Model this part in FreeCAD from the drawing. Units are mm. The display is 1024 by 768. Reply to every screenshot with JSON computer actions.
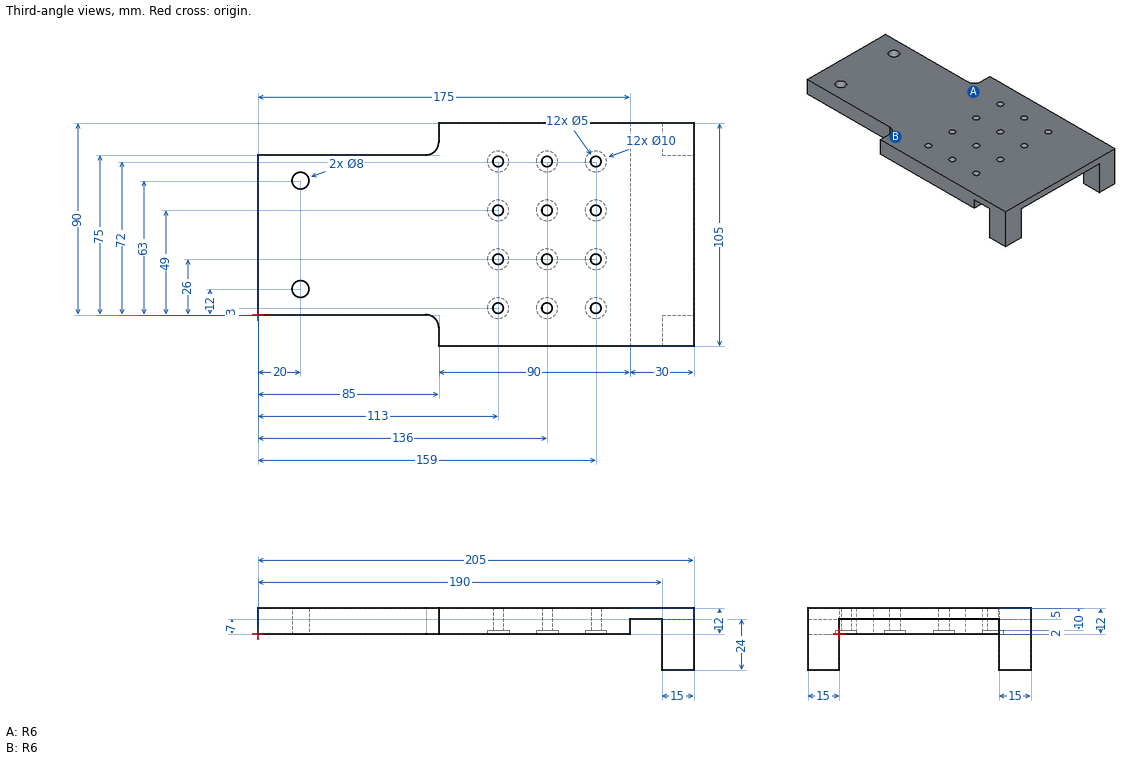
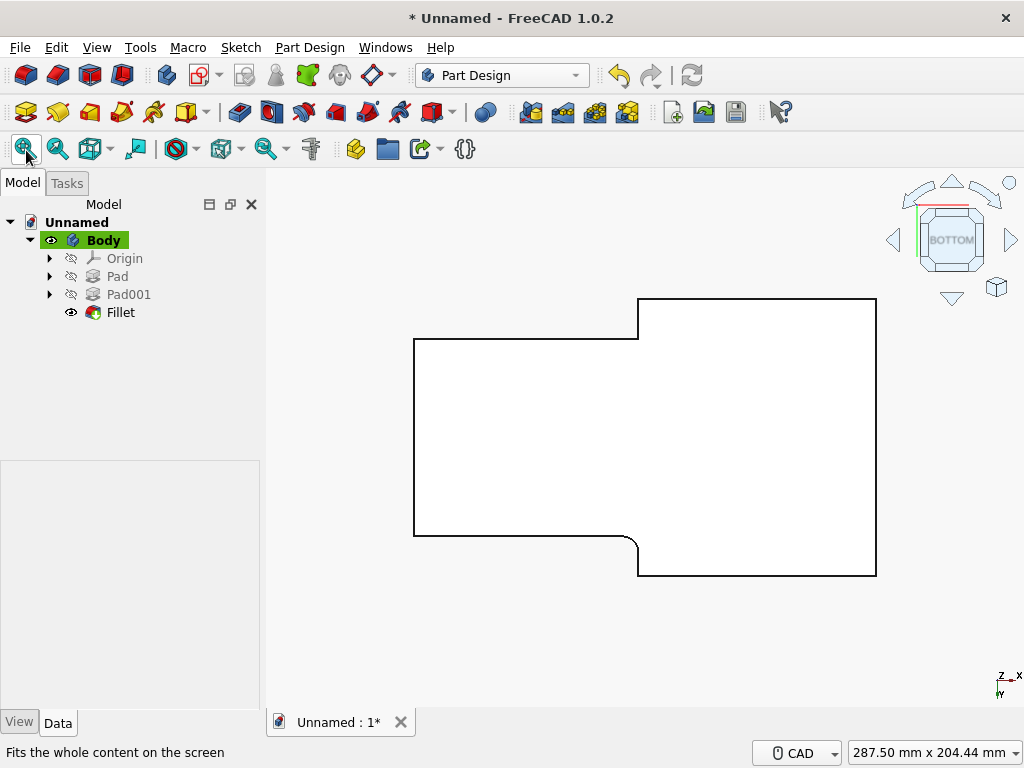
{"action": "key", "text": "4"}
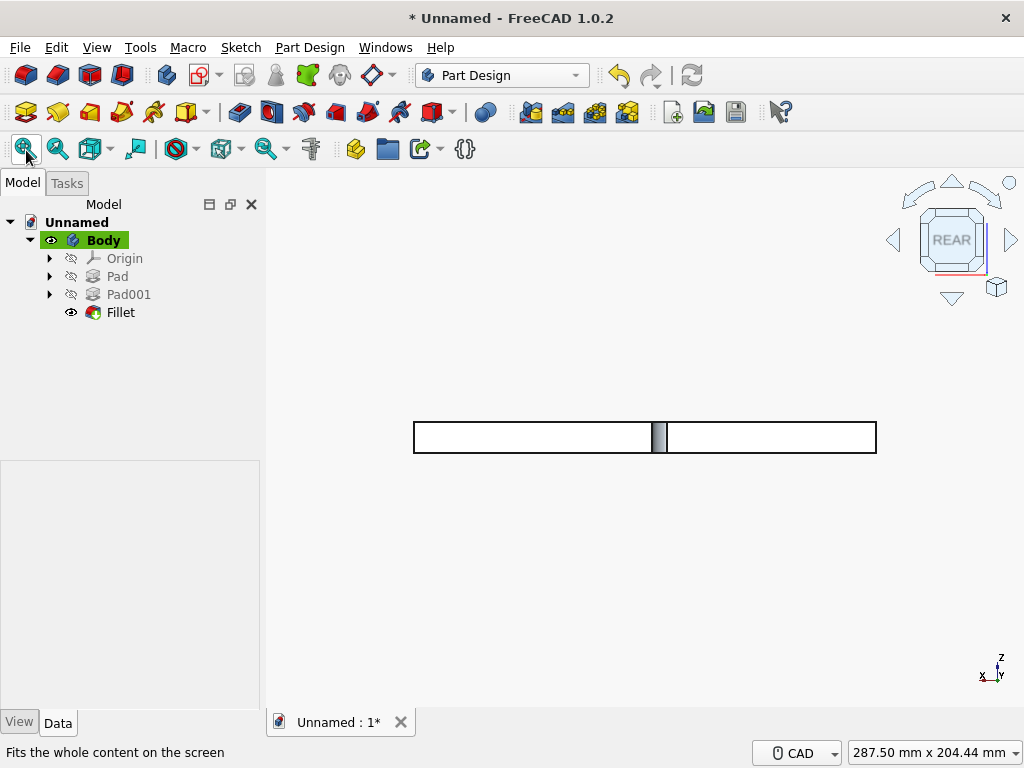
{"action": "key", "text": "6"}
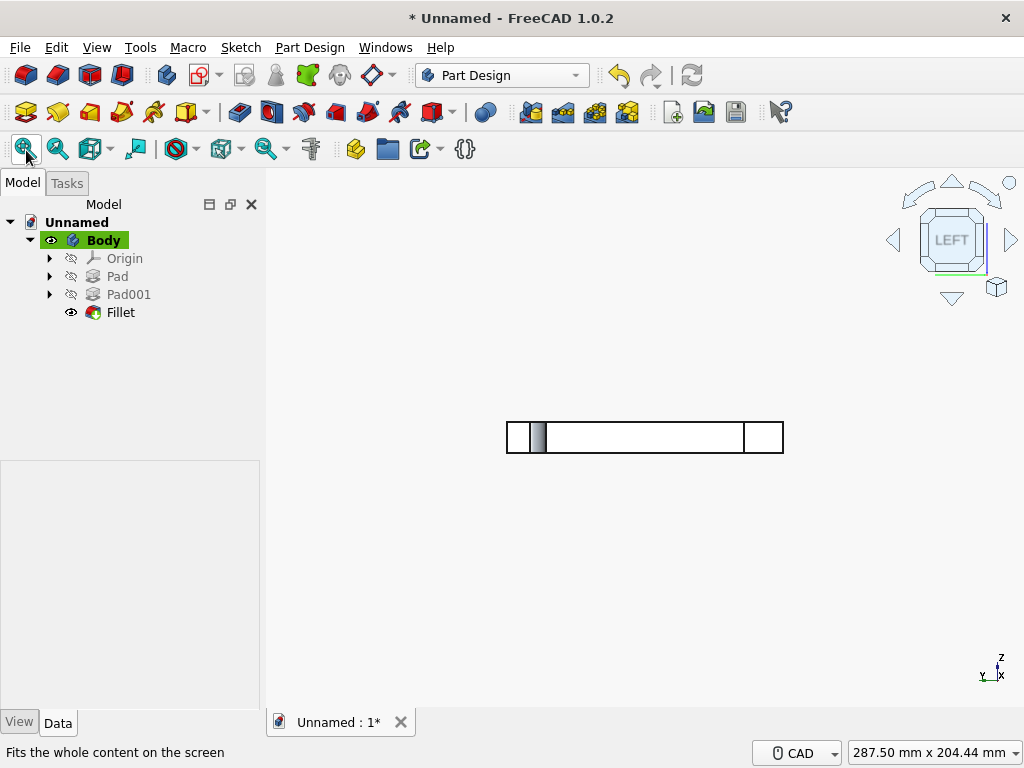
{"action": "left_click", "coordinate": [26, 150]}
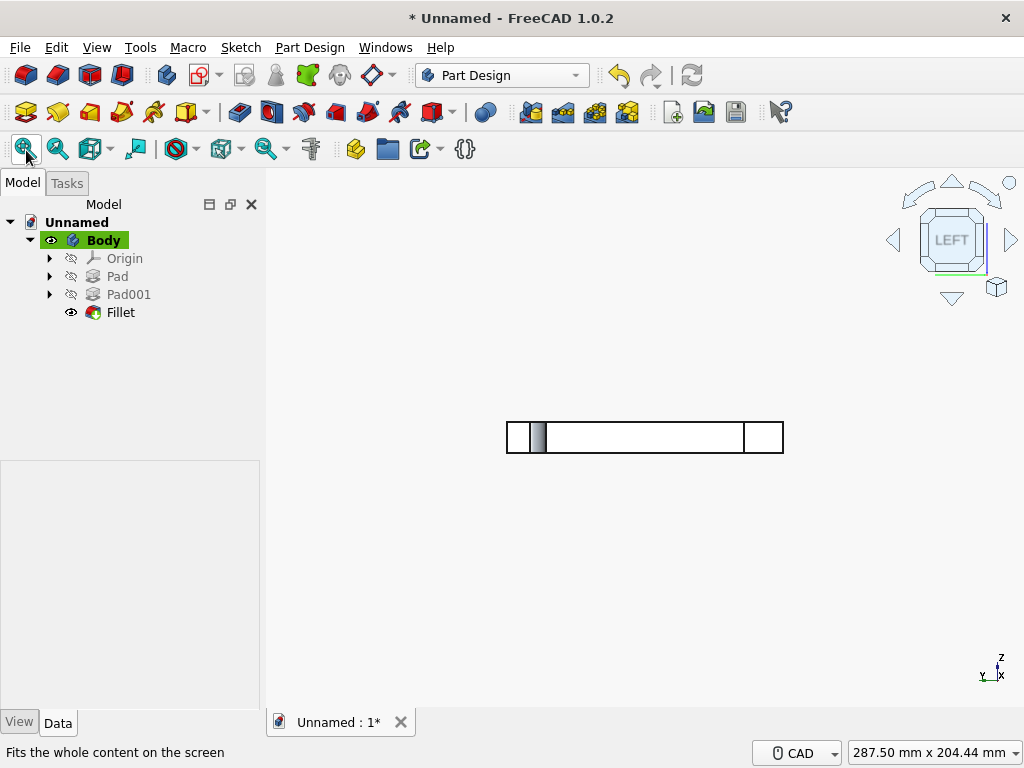
{"action": "key", "text": "v 3"}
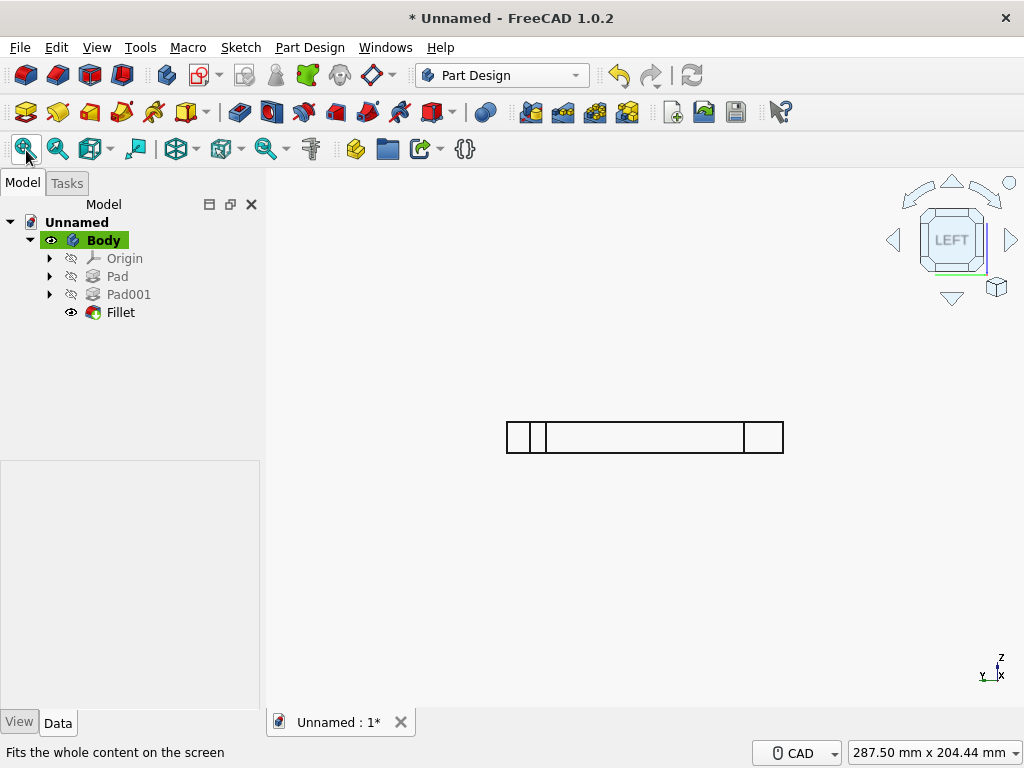
{"action": "key", "text": "0"}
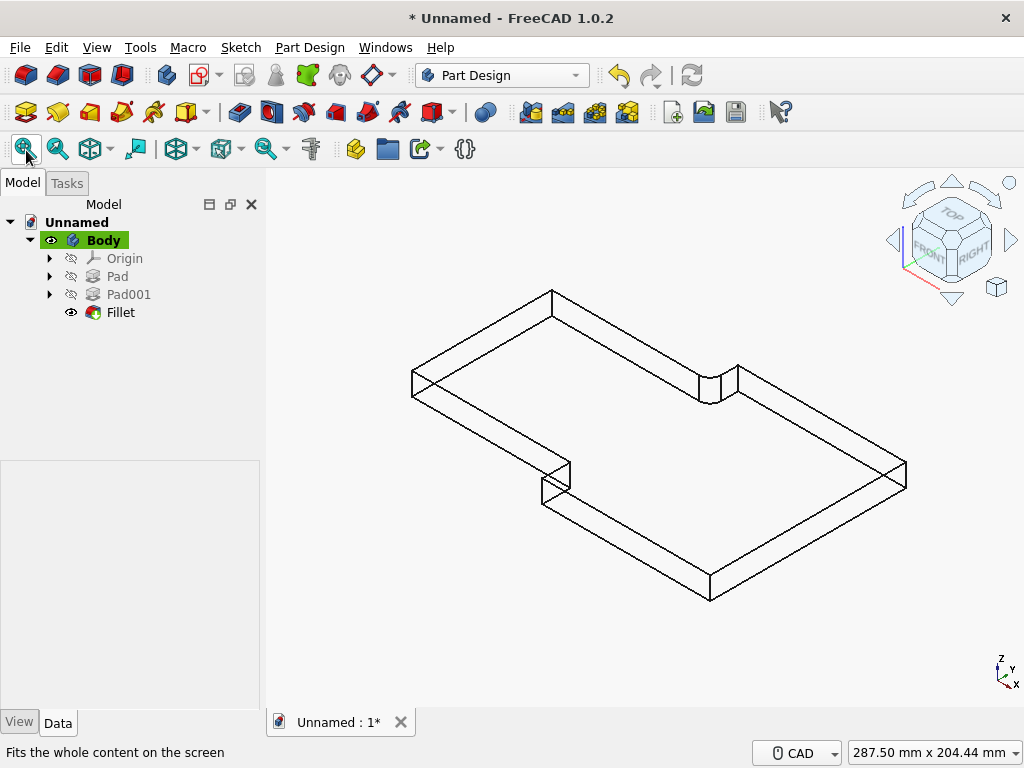
{"action": "left_click", "coordinate": [570, 474]}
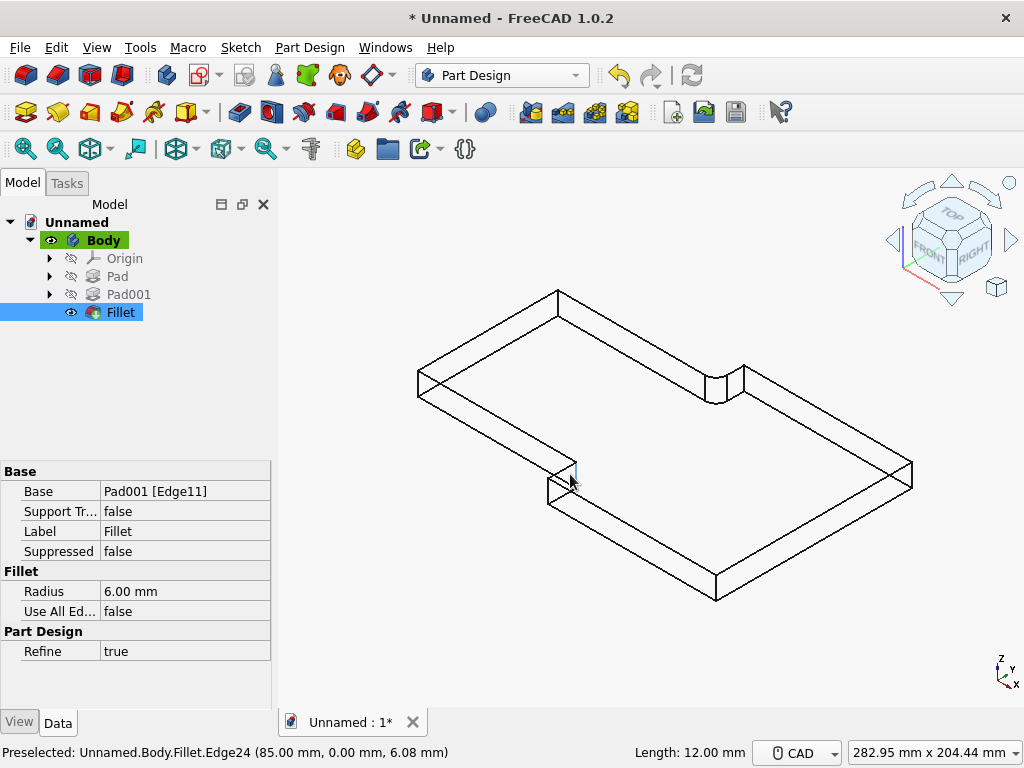
{"action": "key", "text": "v 1"}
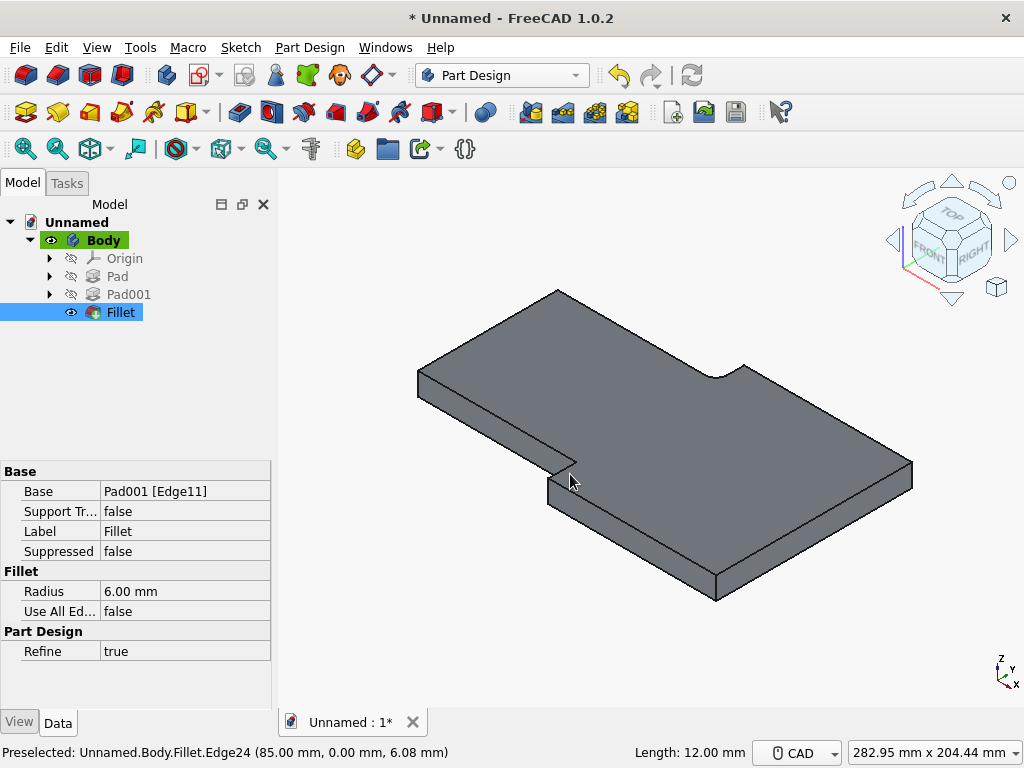
{"action": "left_click", "coordinate": [26, 76]}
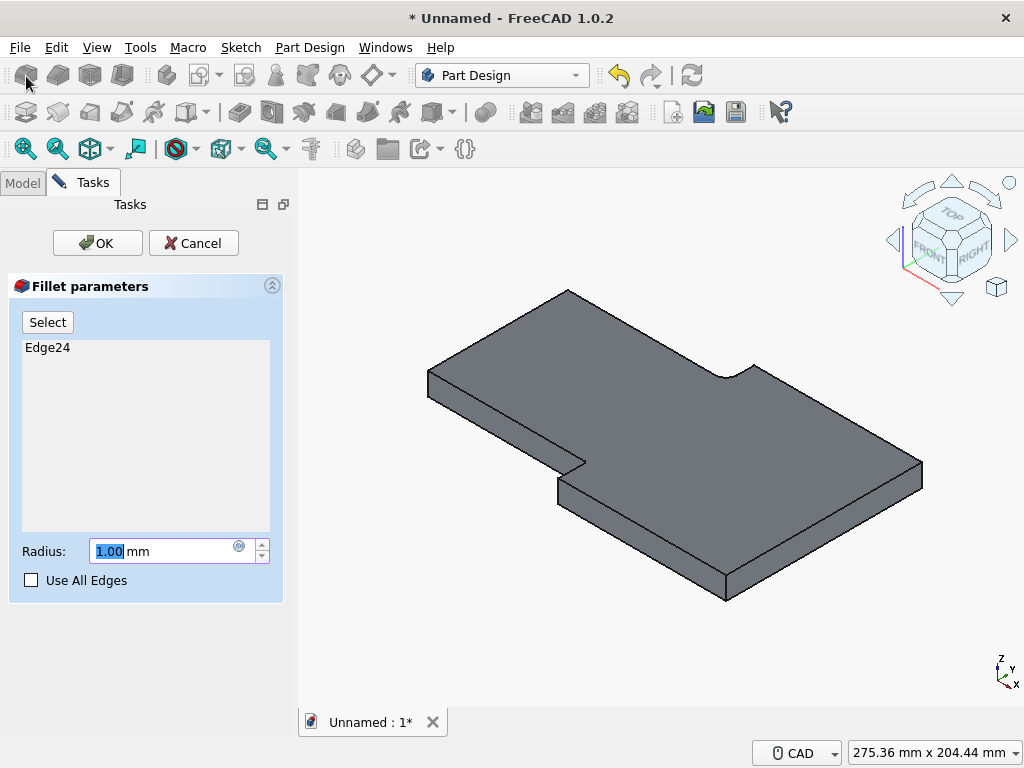
{"action": "type", "text": "6"}
{"action": "key", "text": "Tab"}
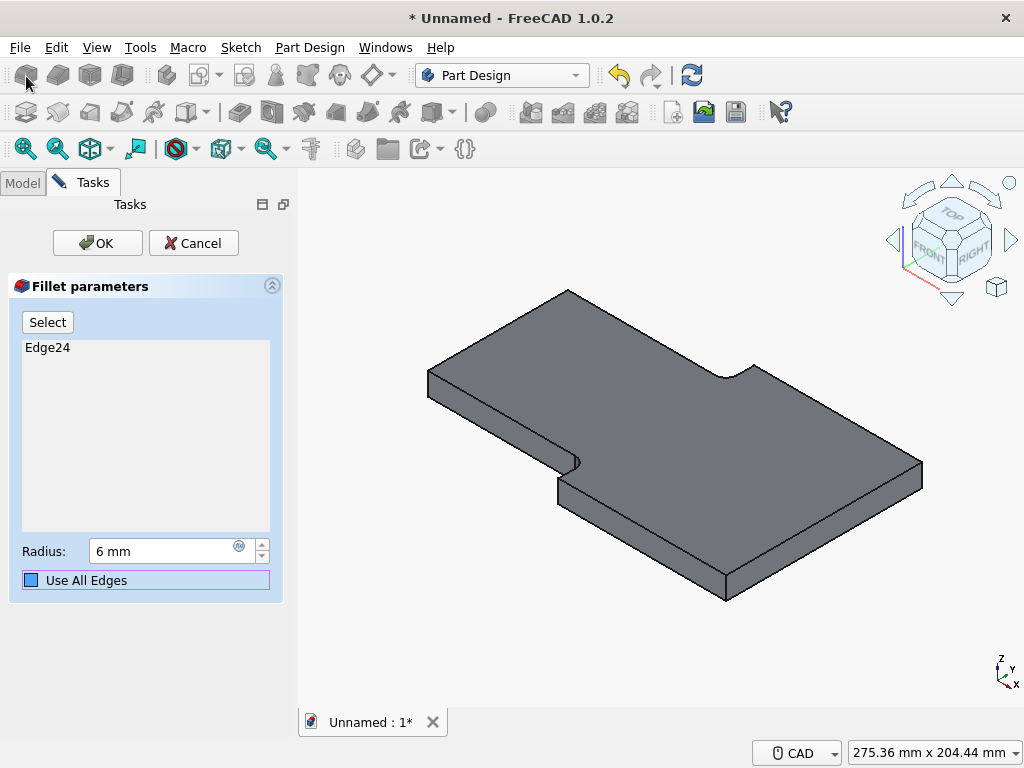
{"action": "left_click", "coordinate": [98, 243]}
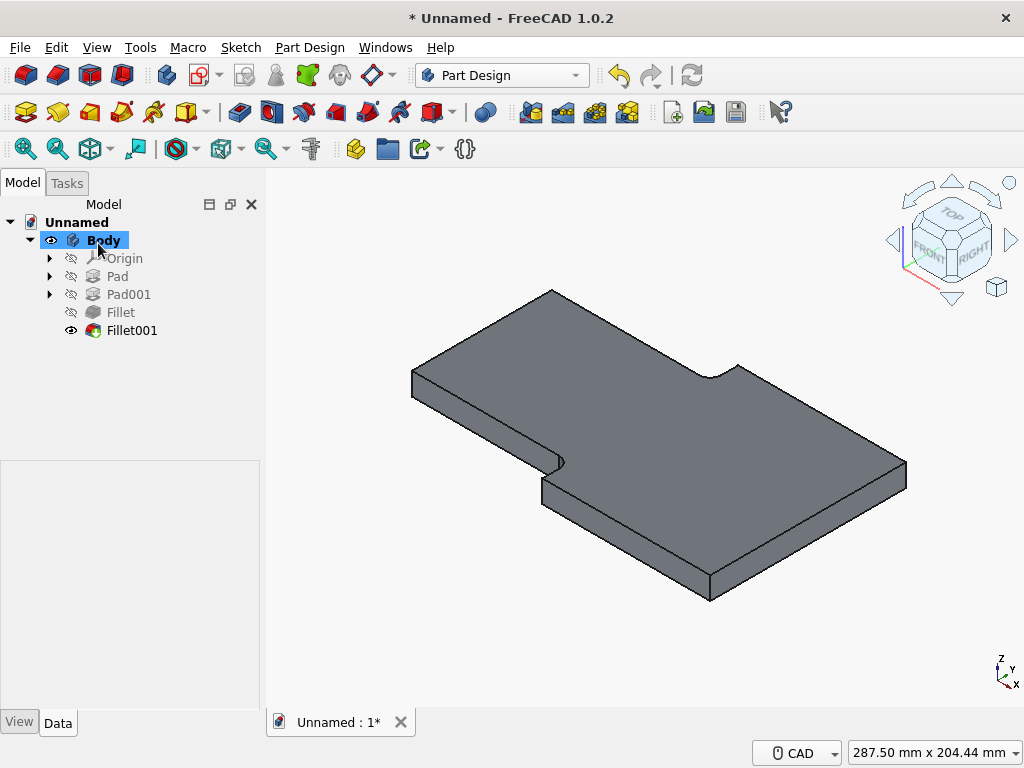
{"action": "left_click", "coordinate": [692, 450]}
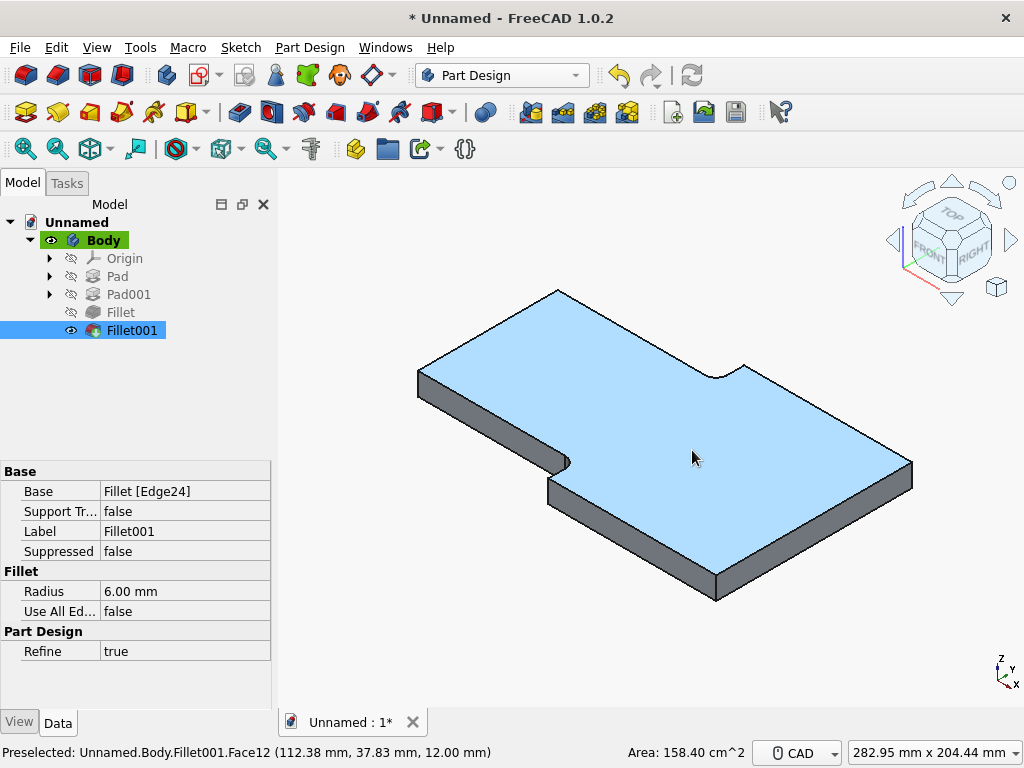
{"action": "left_click", "coordinate": [200, 76]}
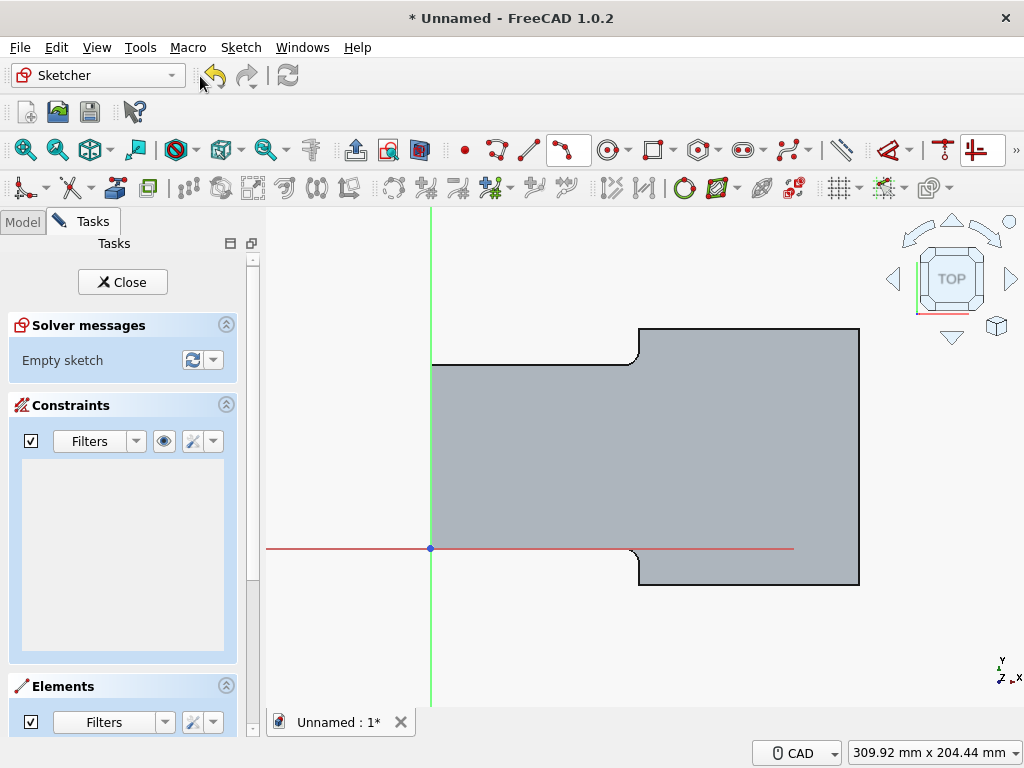
{"action": "scroll", "coordinate": [294, 457], "scroll_direction": "down", "scroll_amount": 1}